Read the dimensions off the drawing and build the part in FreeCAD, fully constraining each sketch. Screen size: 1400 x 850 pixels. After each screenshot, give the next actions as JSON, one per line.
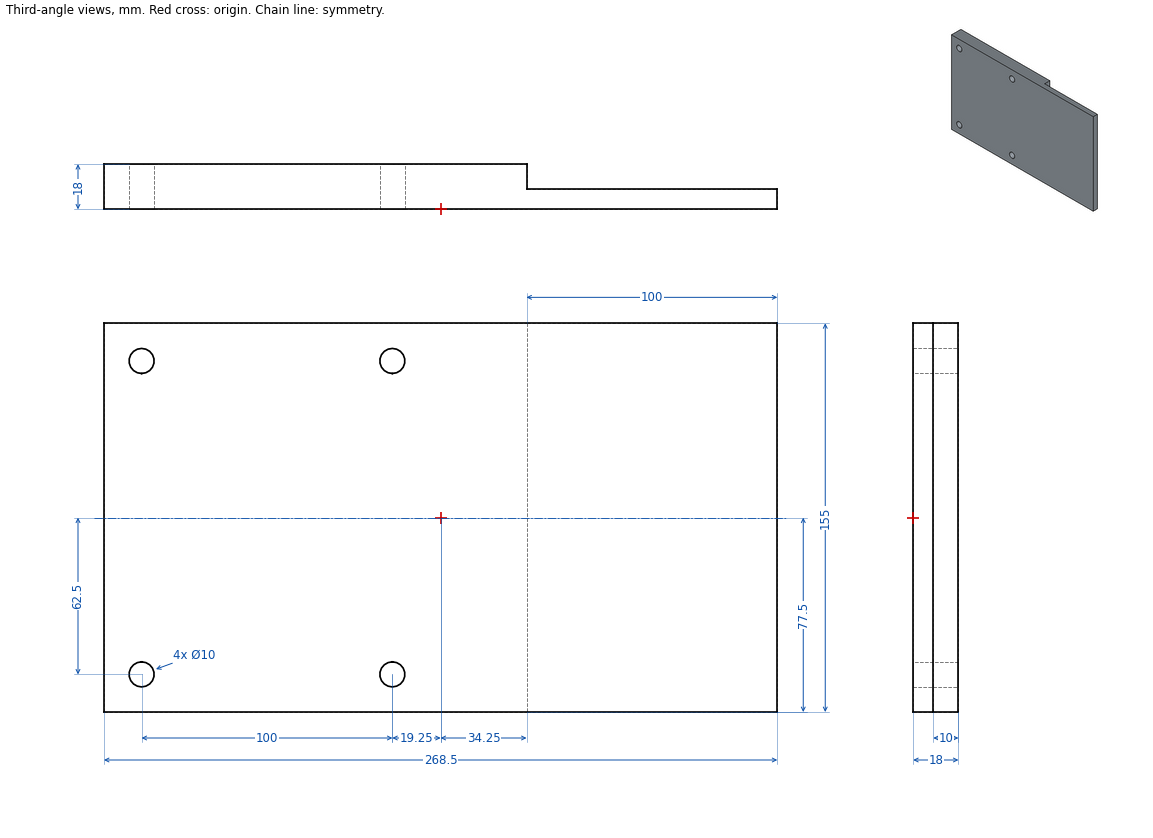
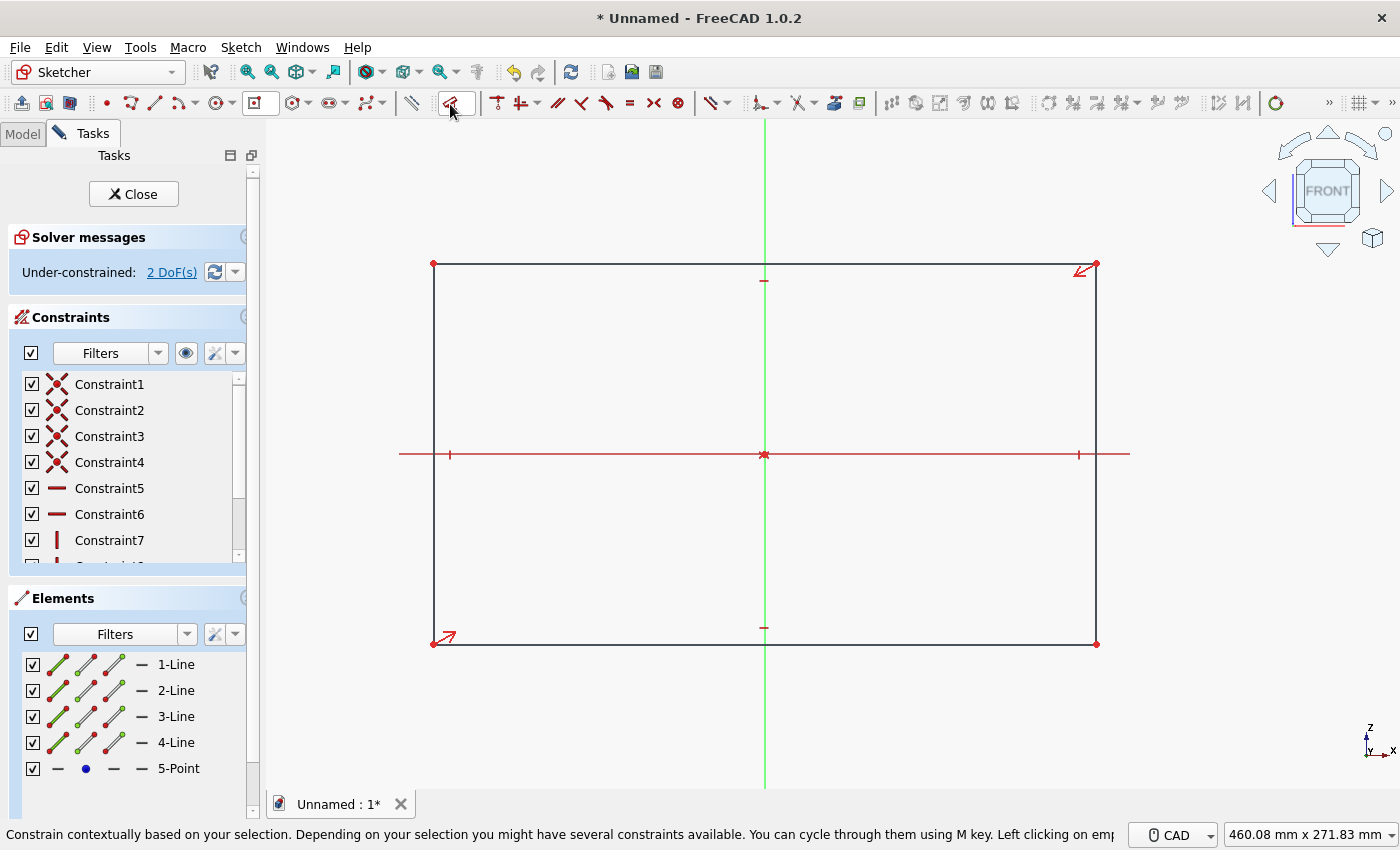
{"action": "left_click", "coordinate": [1096, 530]}
{"action": "left_click", "coordinate": [1130, 367]}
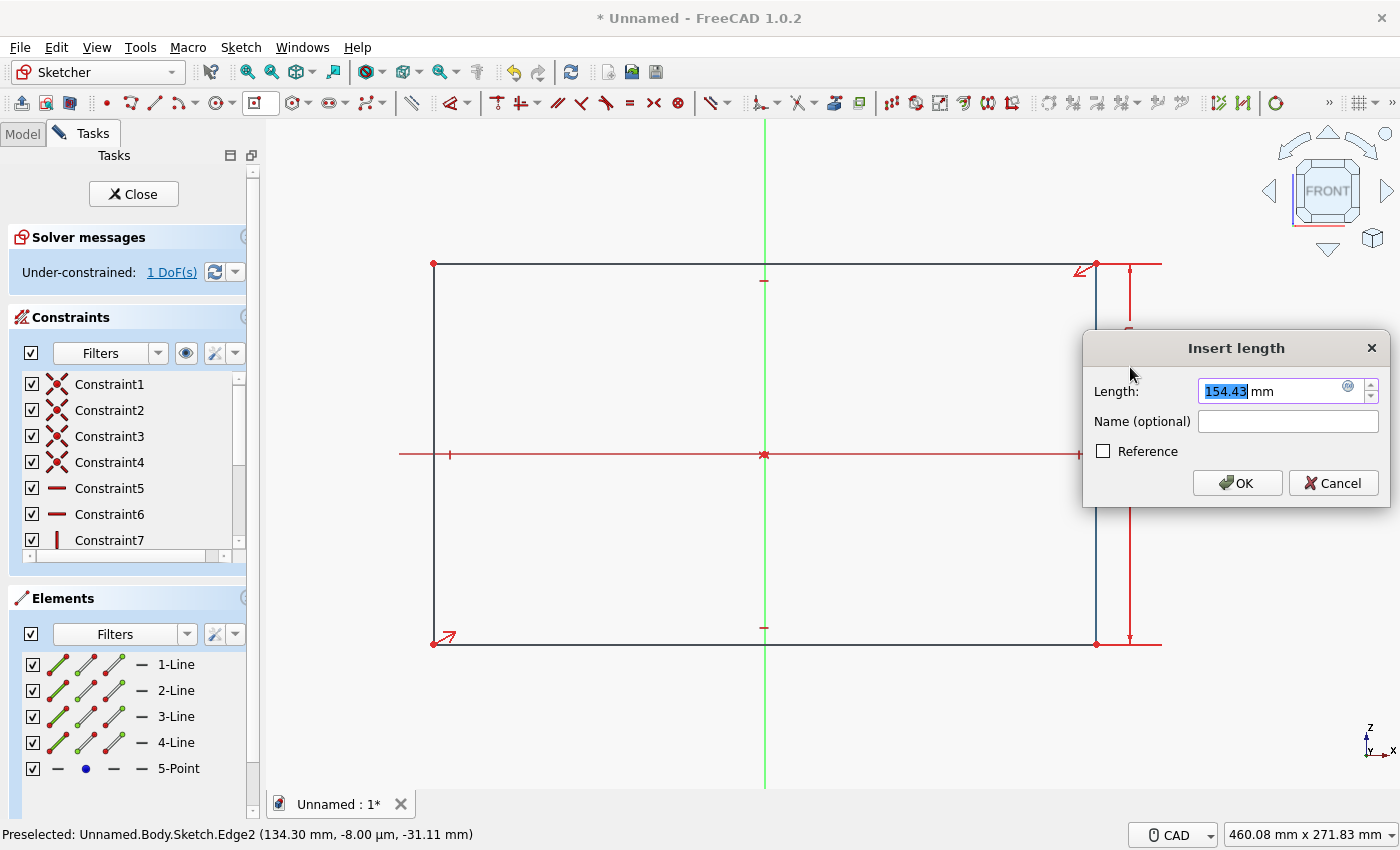
{"action": "type", "text": "155"}
{"action": "key", "text": "Return"}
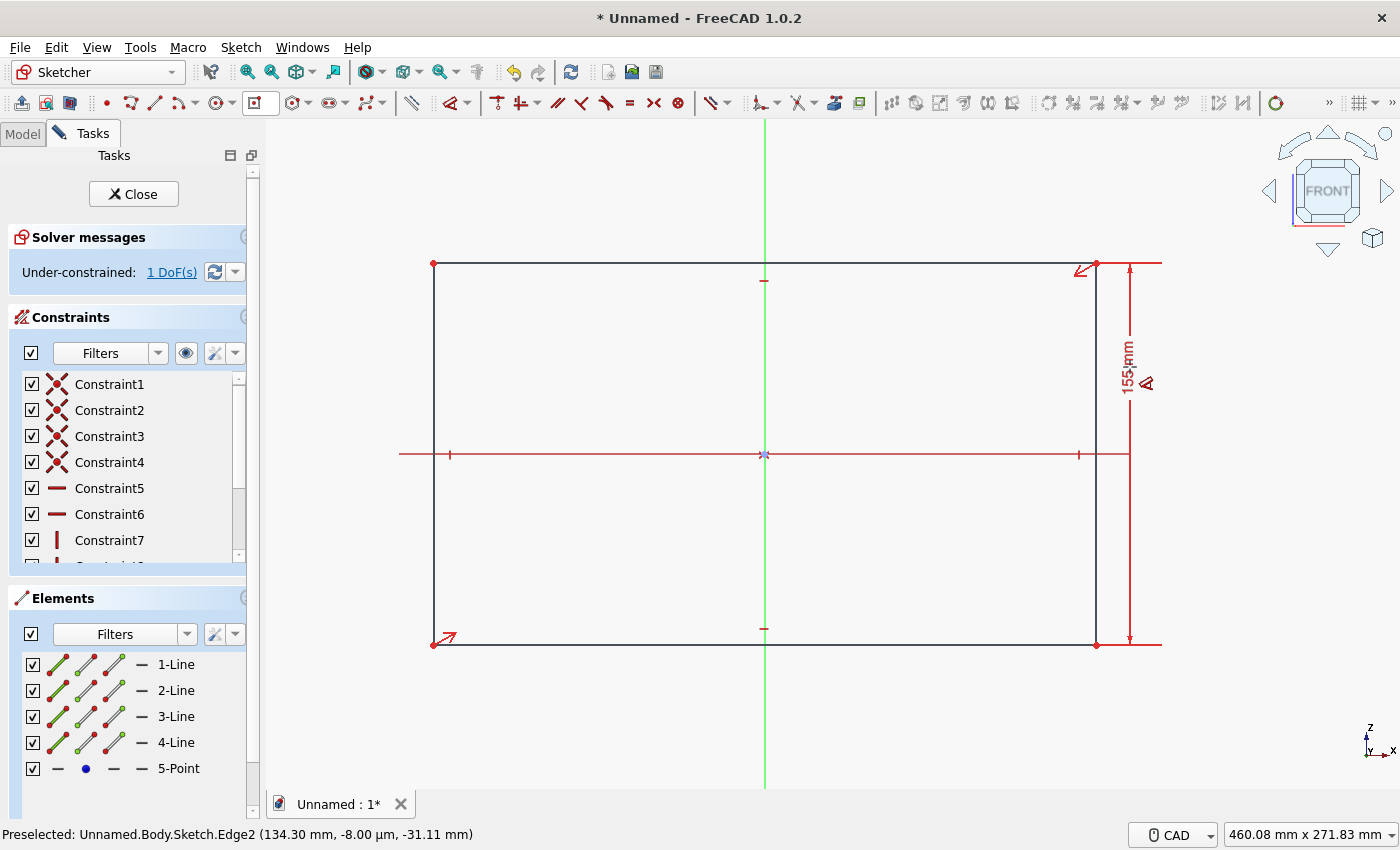
{"action": "left_click", "coordinate": [633, 645]}
{"action": "left_click", "coordinate": [613, 679]}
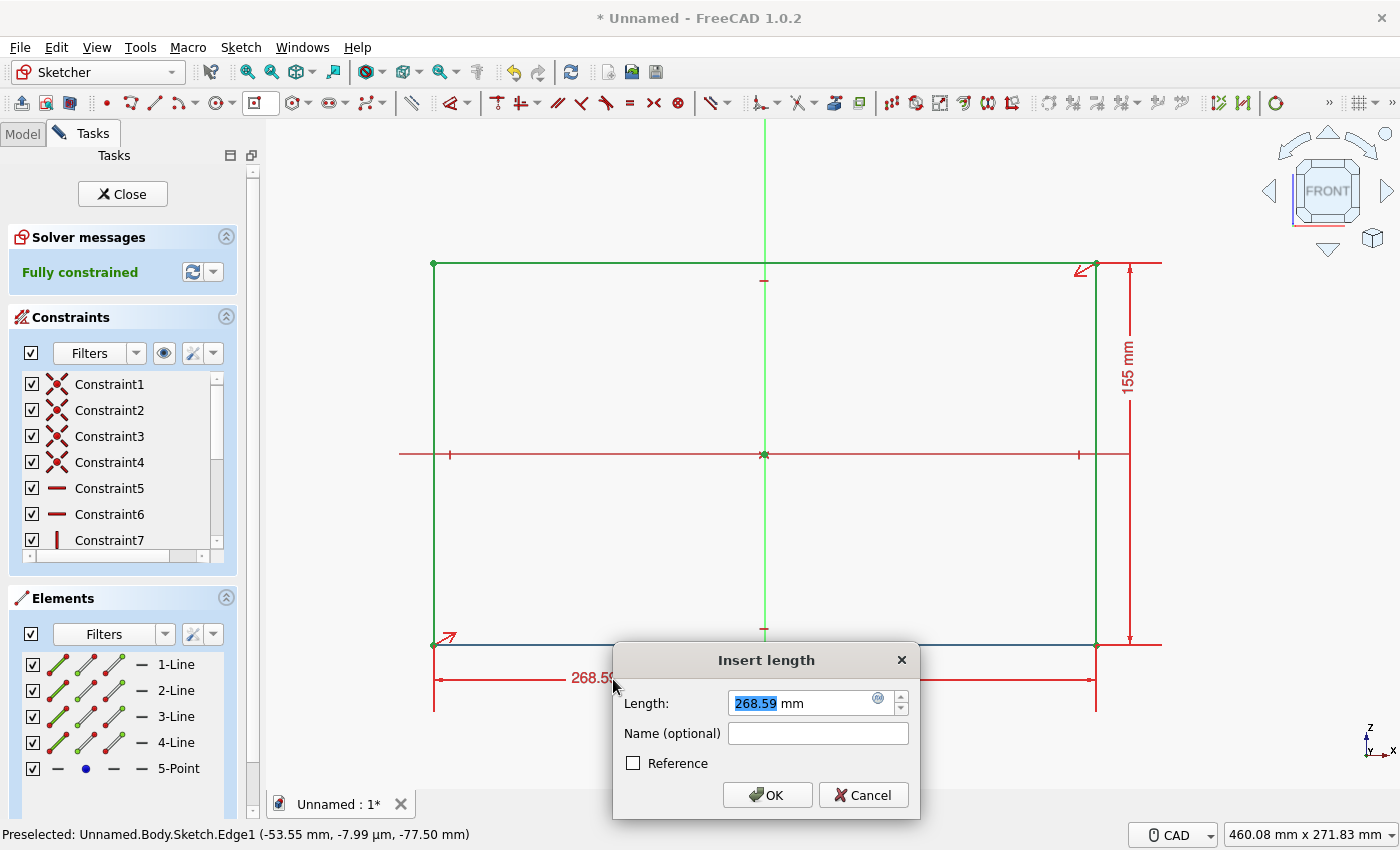
{"action": "type", "text": "268.5"}
{"action": "key", "text": "Return"}
{"action": "key", "text": "Escape"}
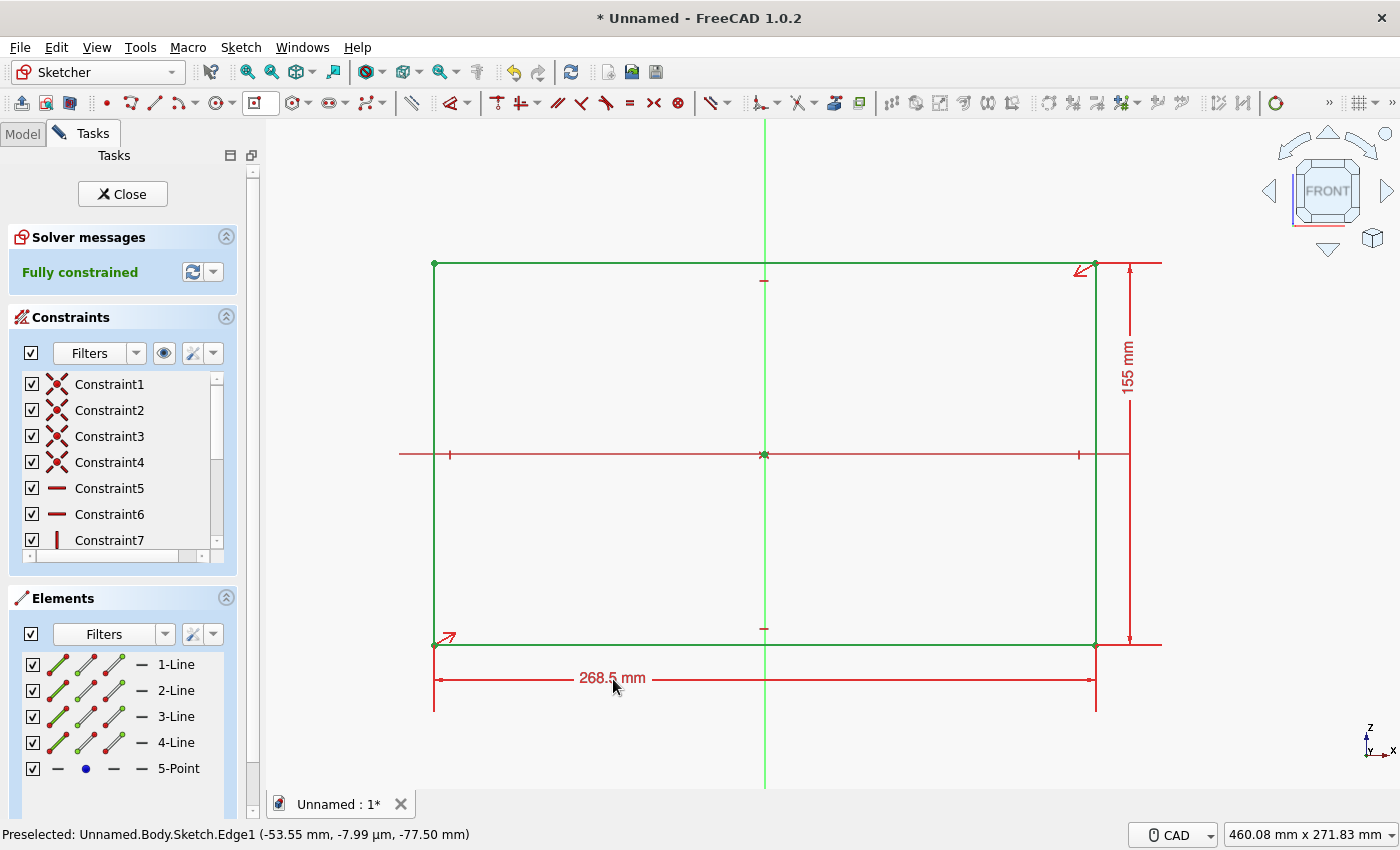
{"action": "left_click", "coordinate": [123, 194]}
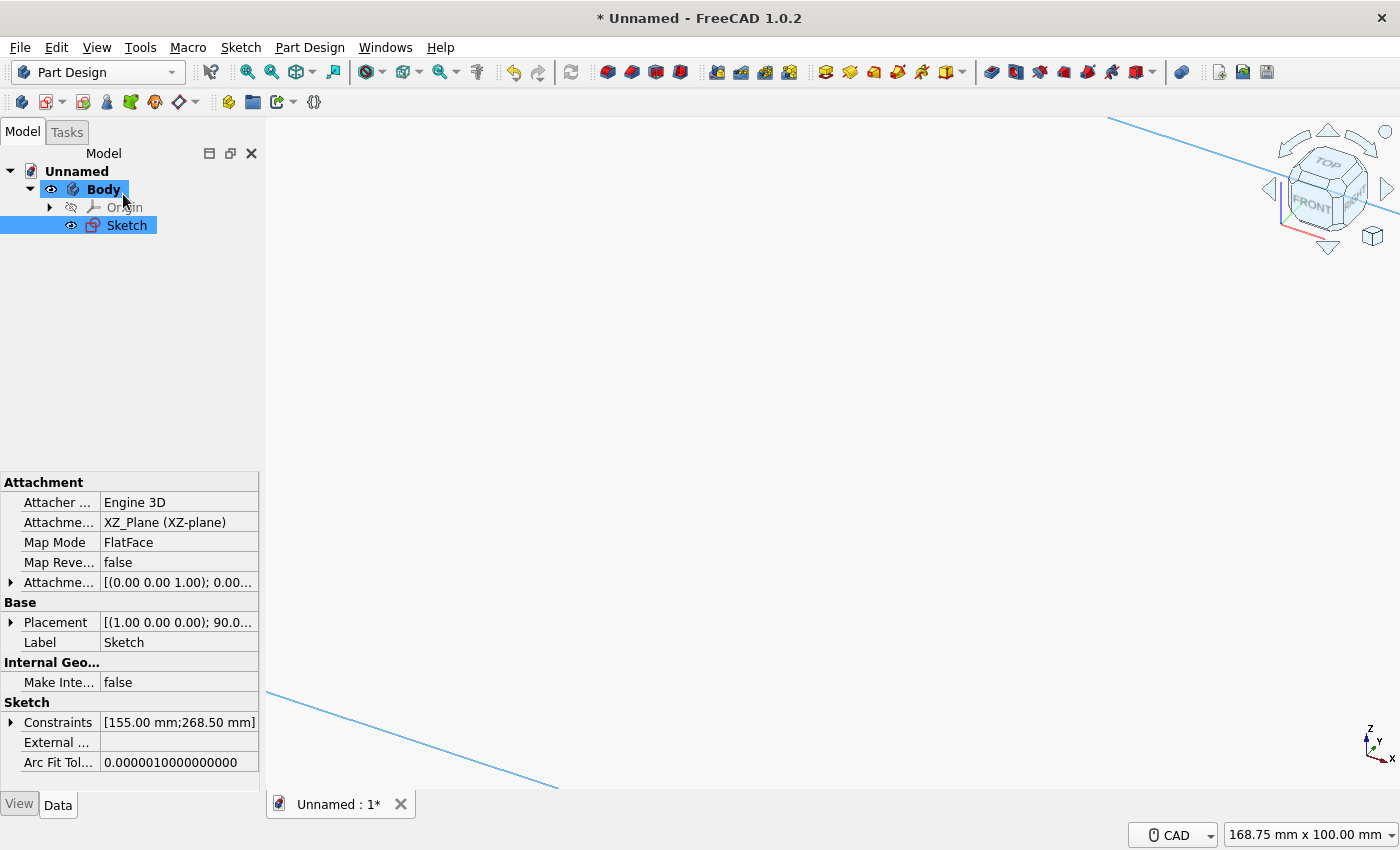
{"action": "left_click", "coordinate": [826, 72]}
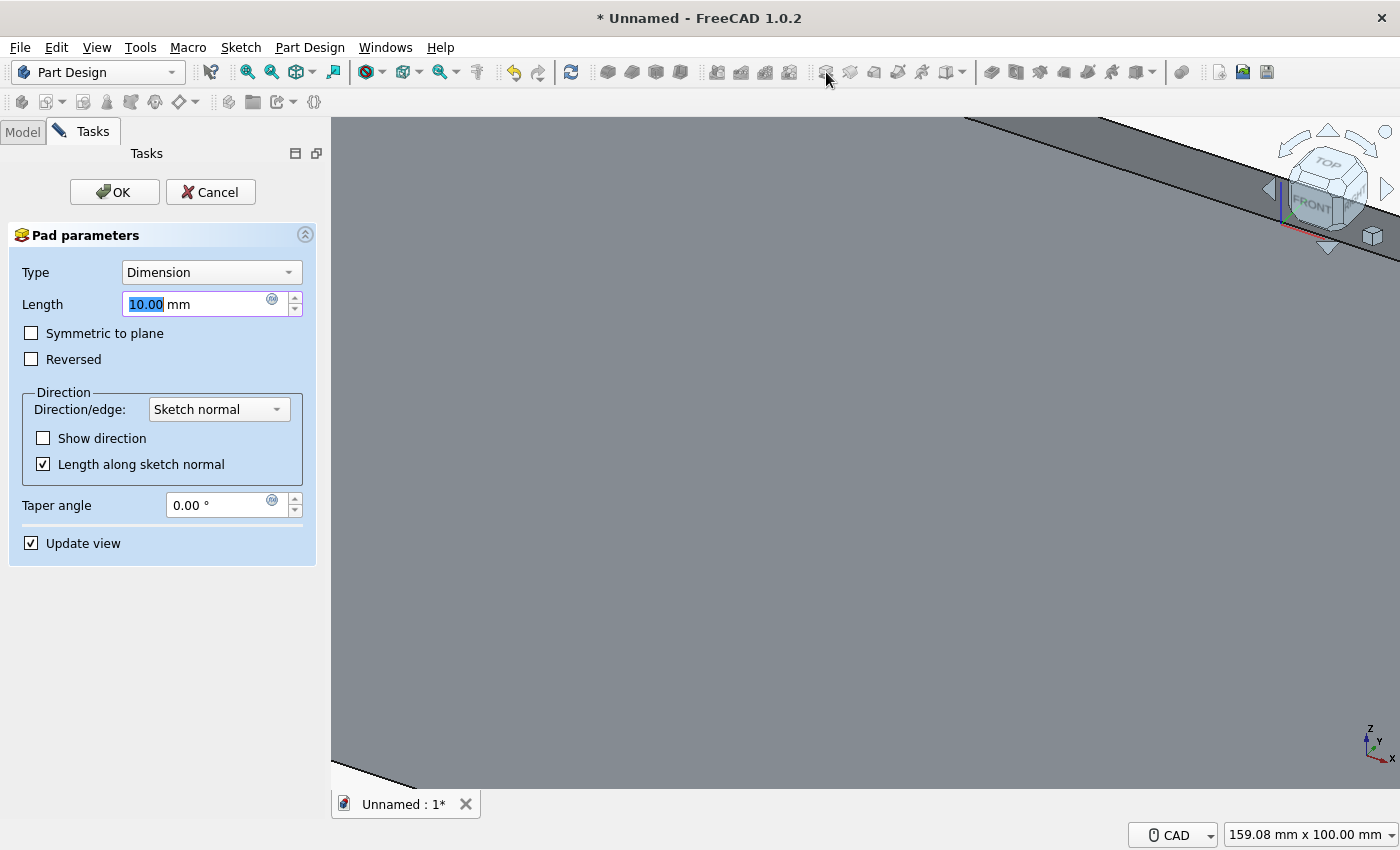
{"action": "type", "text": "18"}
{"action": "key", "text": "Tab"}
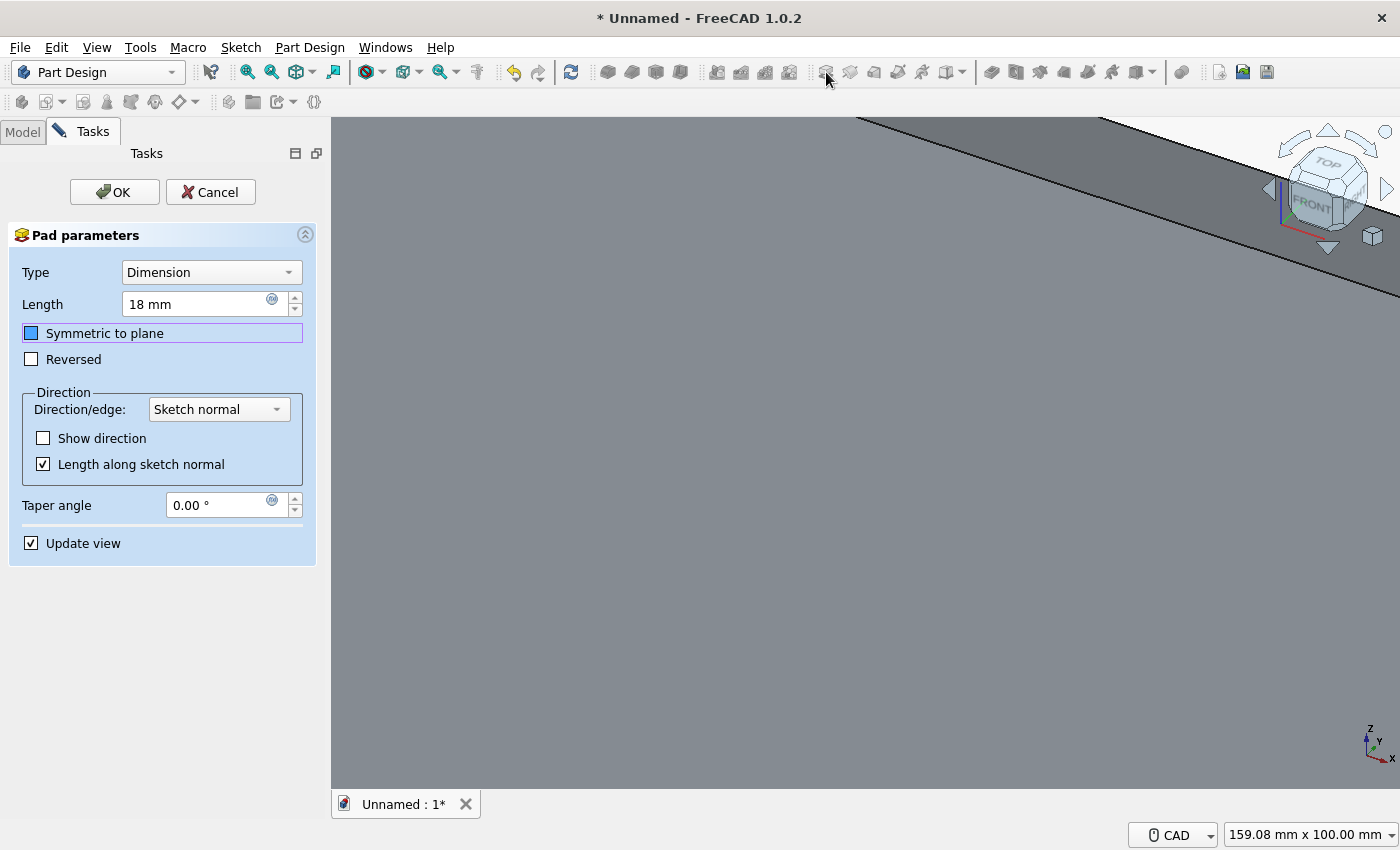
{"action": "left_click", "coordinate": [30, 359]}